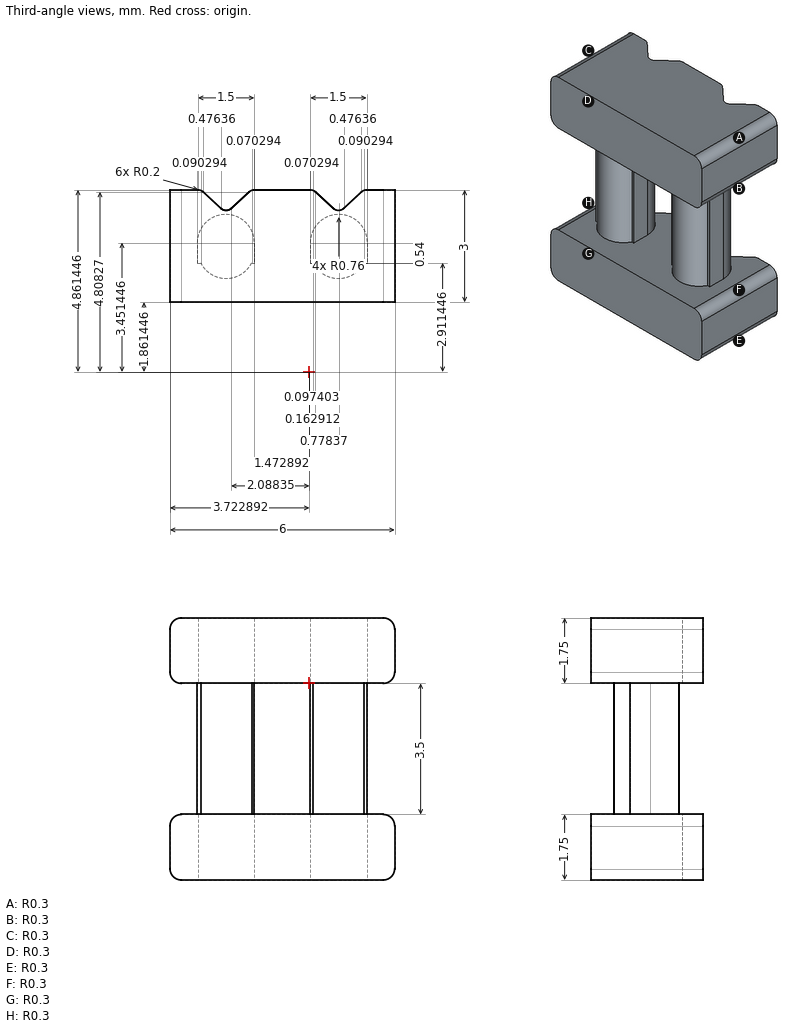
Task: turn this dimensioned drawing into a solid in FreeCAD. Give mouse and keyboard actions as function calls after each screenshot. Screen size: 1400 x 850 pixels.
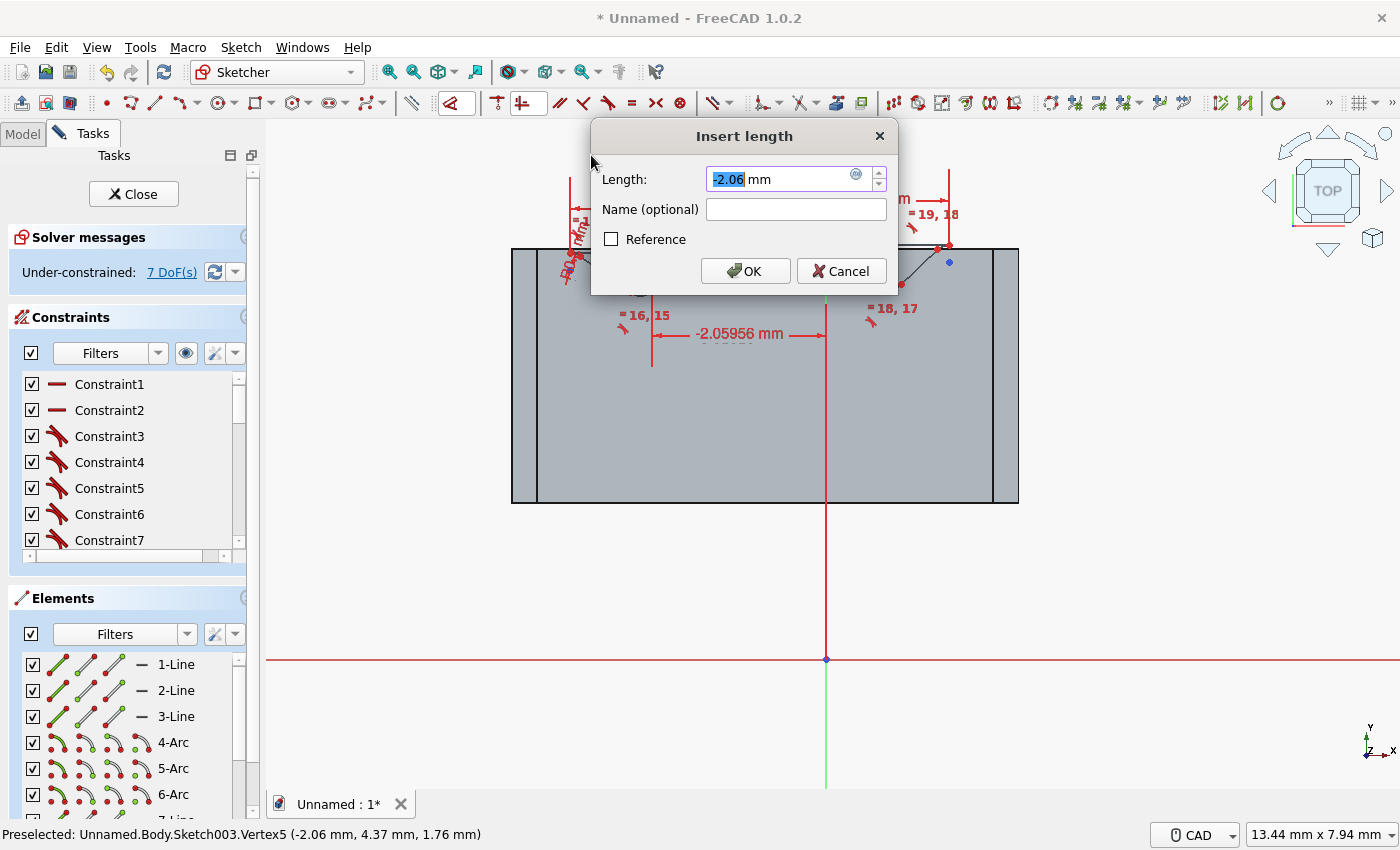
text(-2.08835)
key(Return)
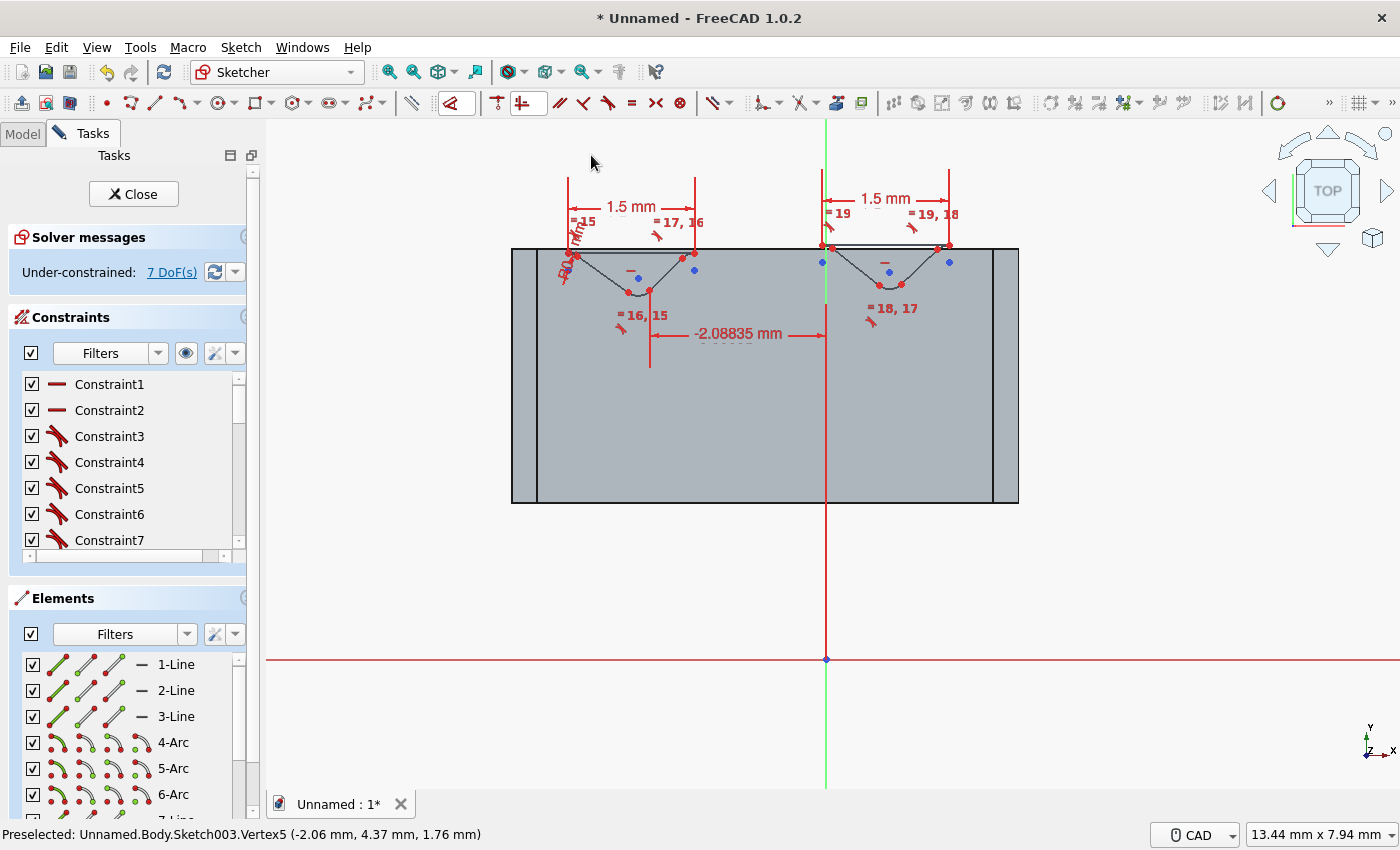
click(683, 258)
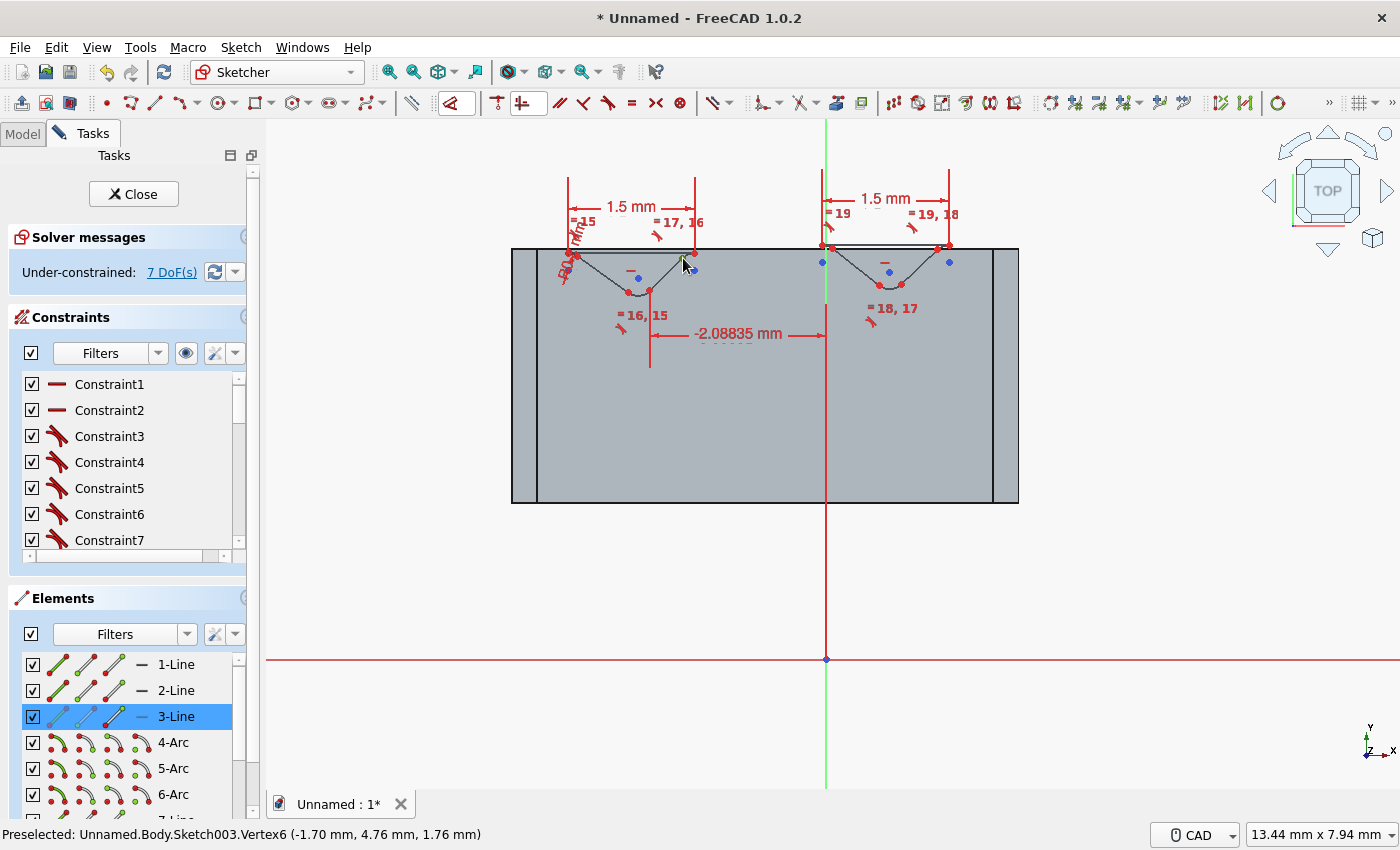
key(i)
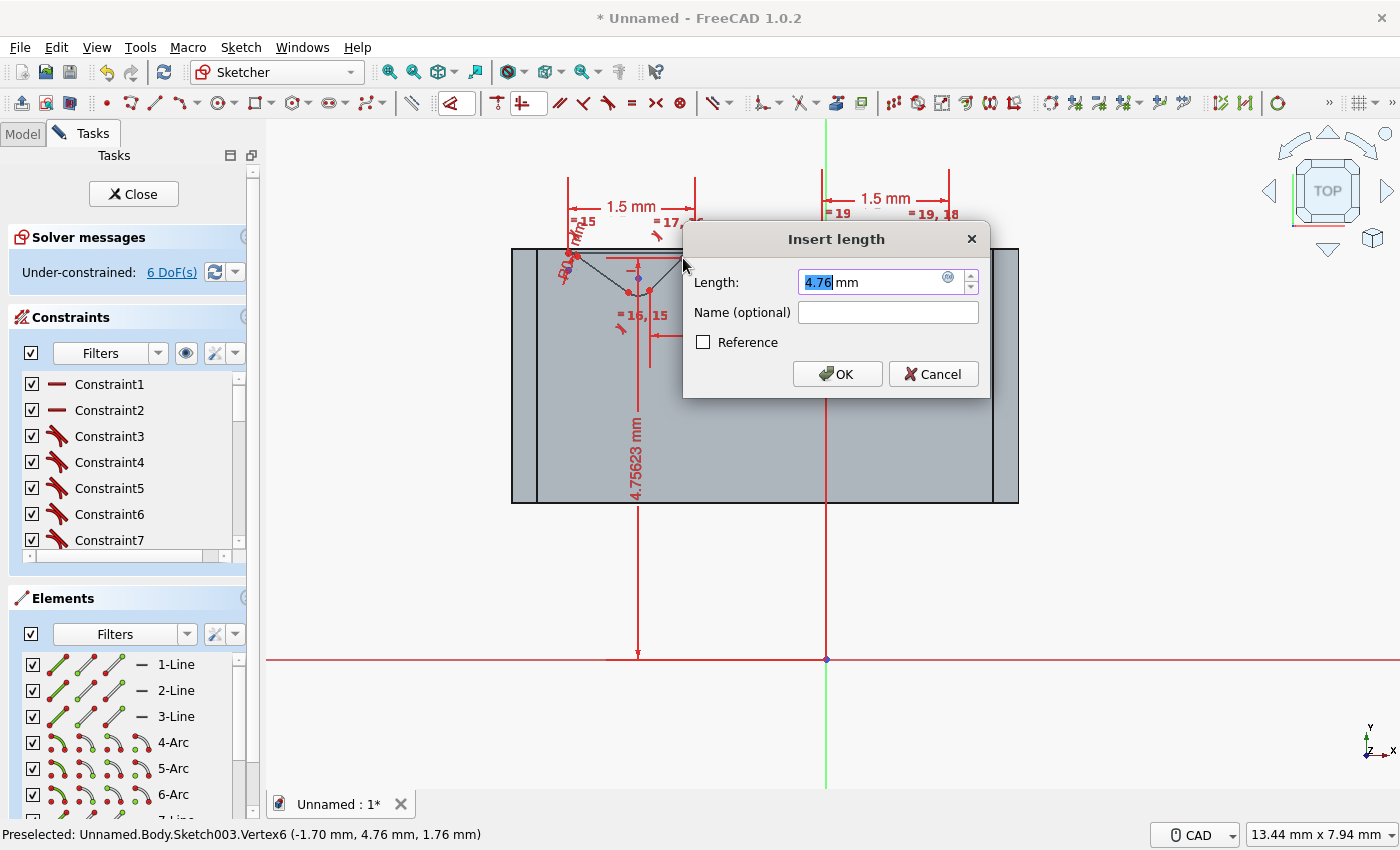
text(4.80827)
key(Return)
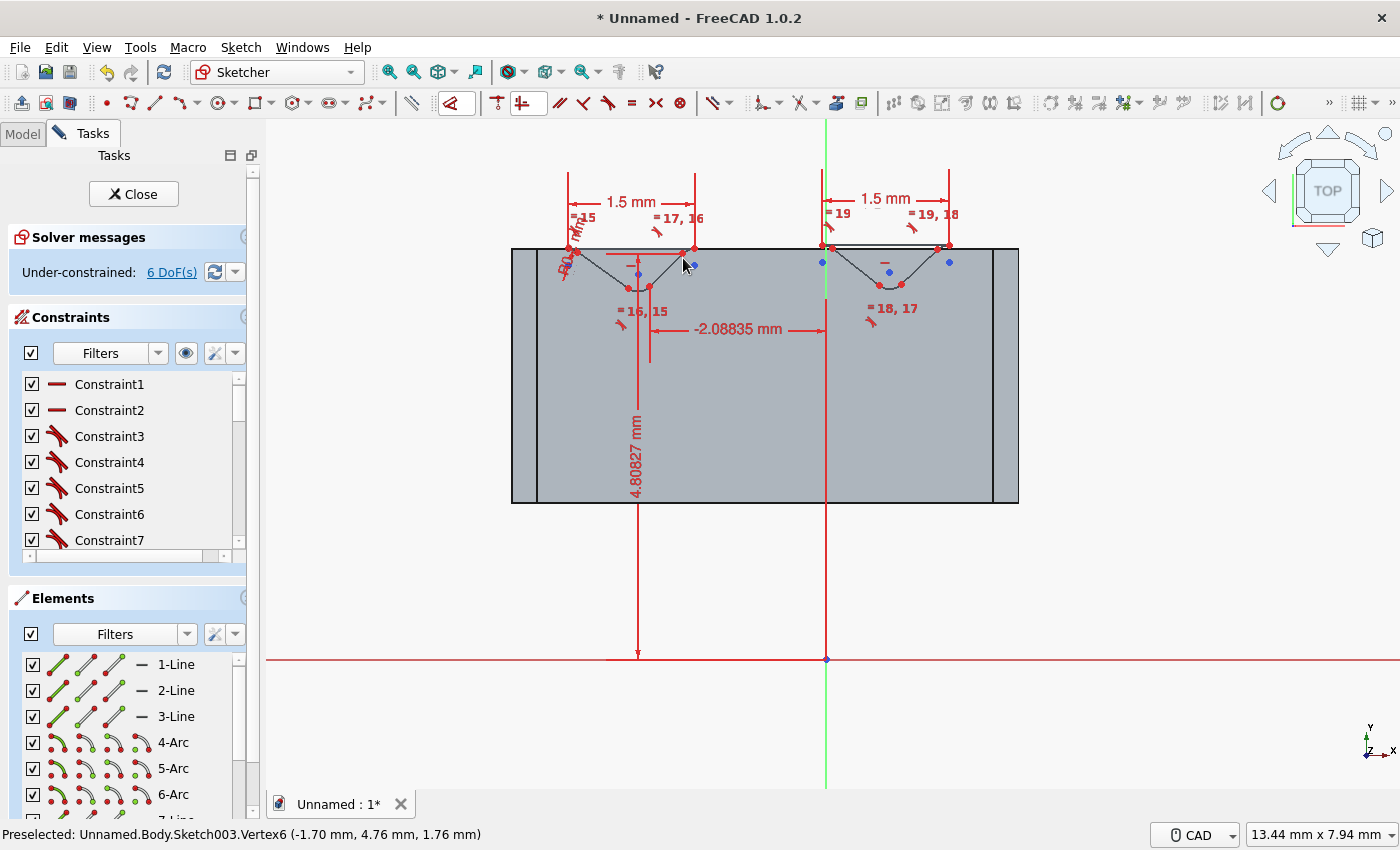
click(833, 249)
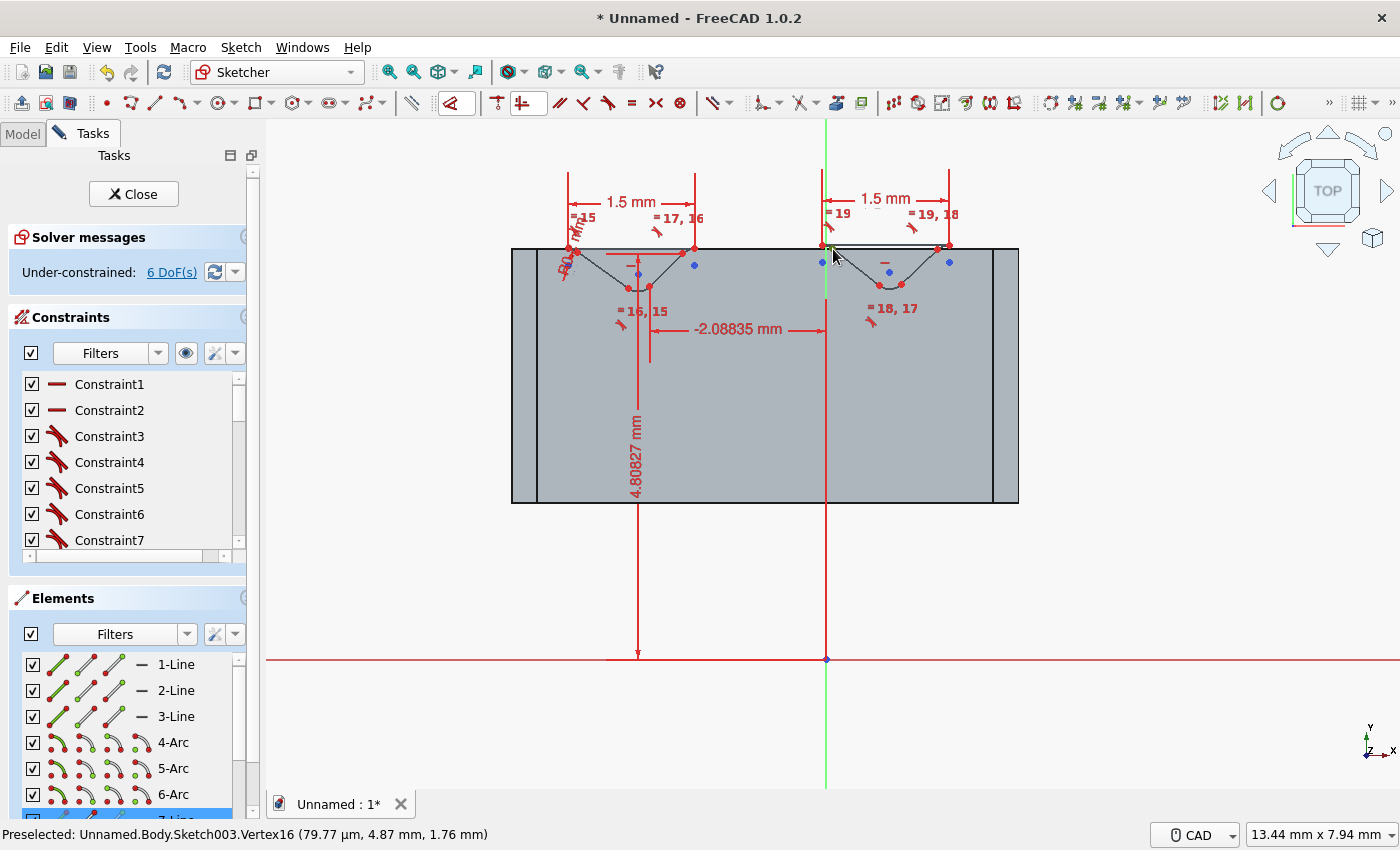
click(470, 104)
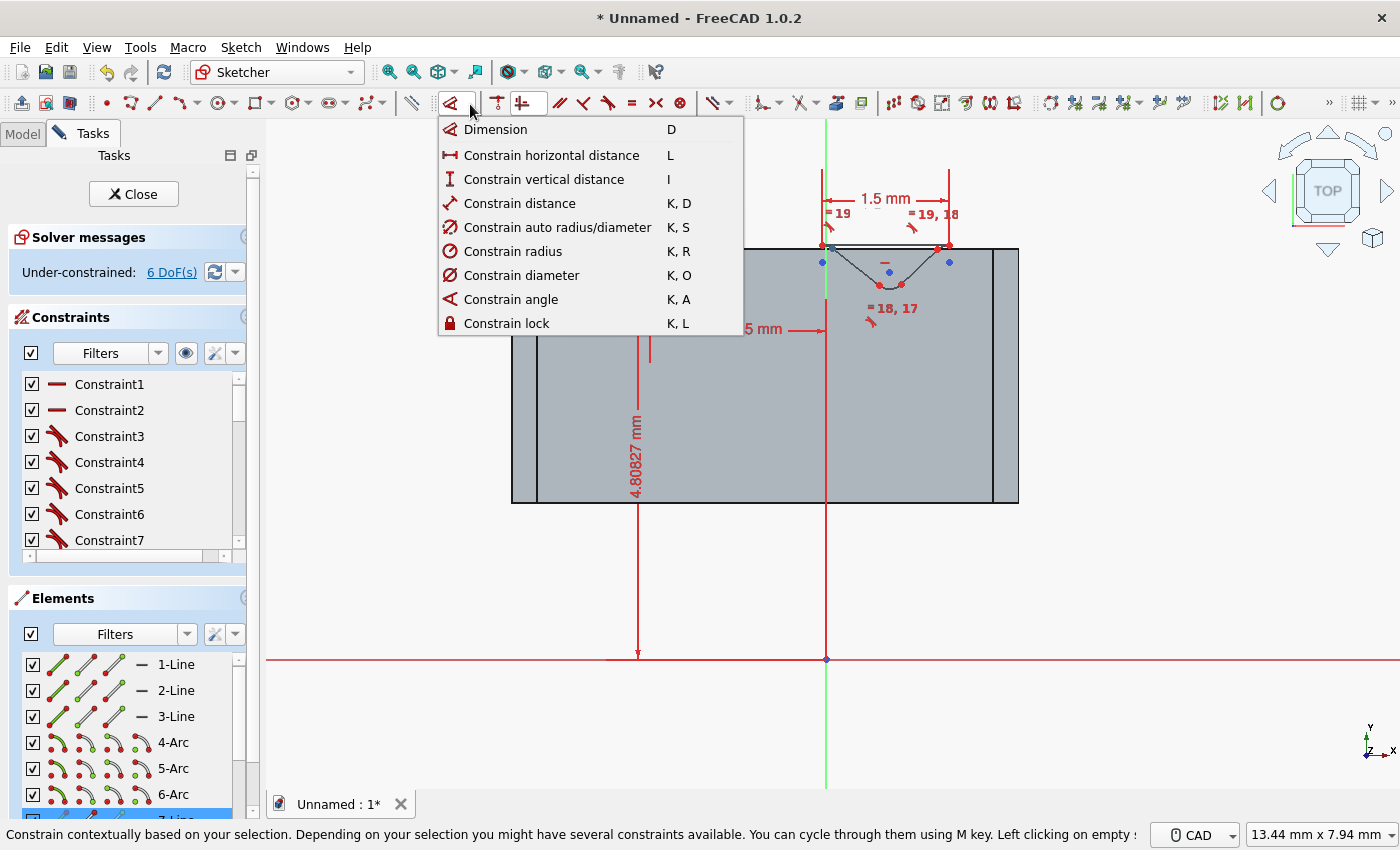
click(591, 179)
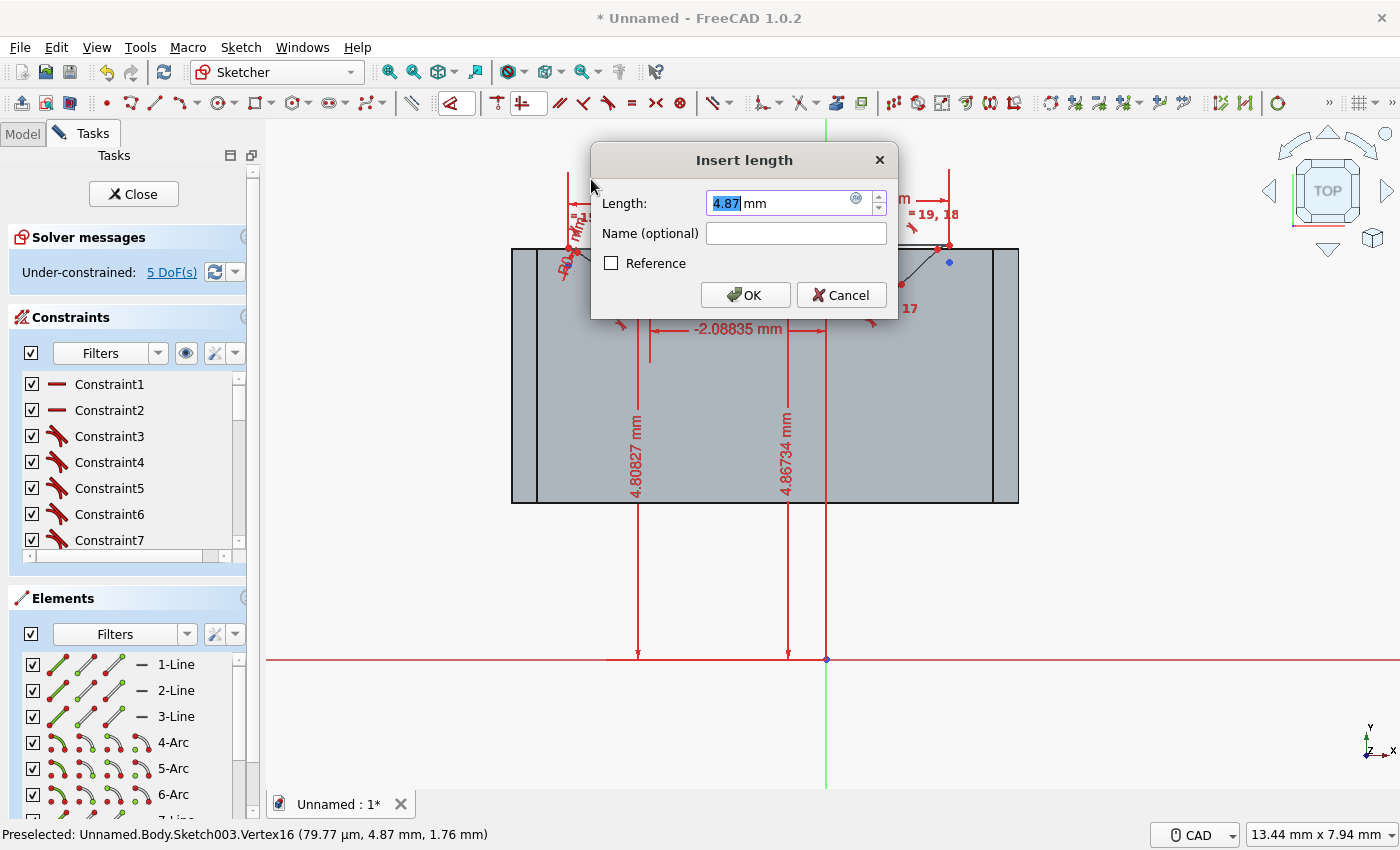
text(4.80827)
key(Return)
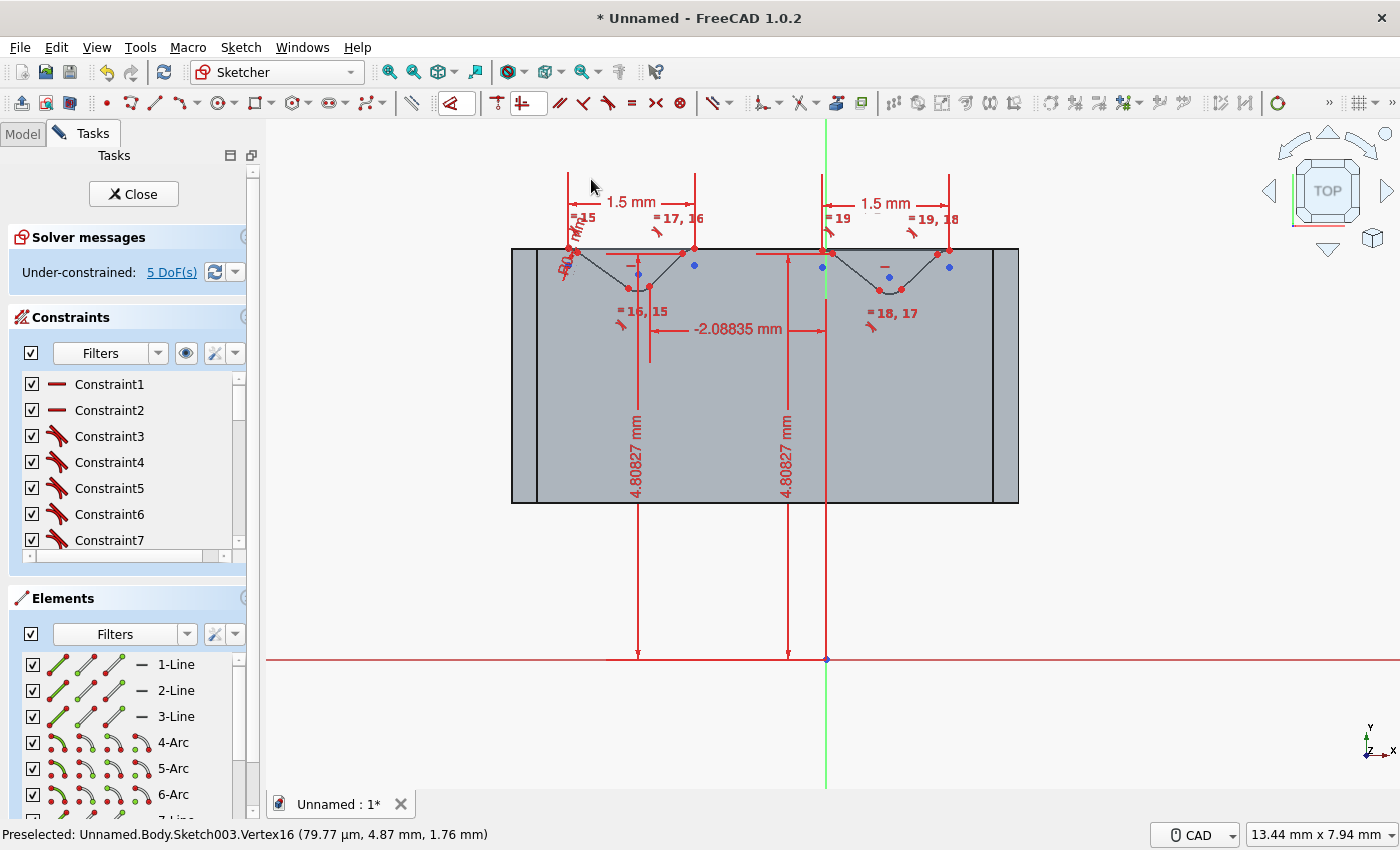
click(593, 263)